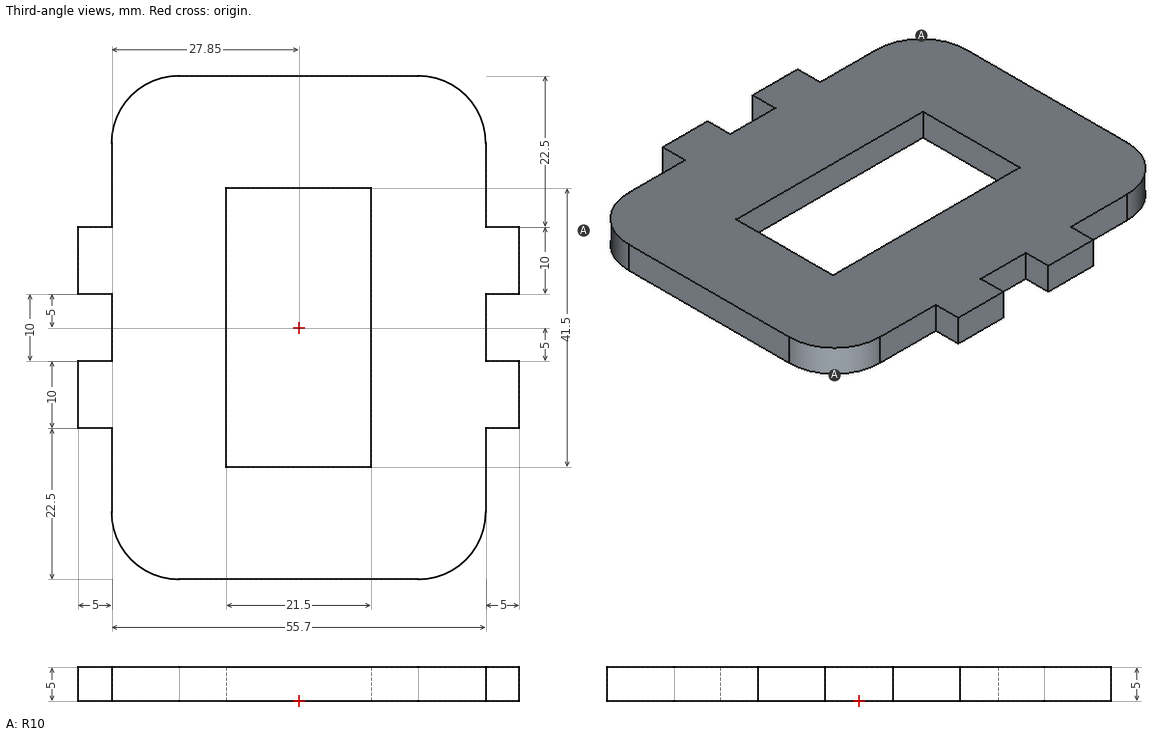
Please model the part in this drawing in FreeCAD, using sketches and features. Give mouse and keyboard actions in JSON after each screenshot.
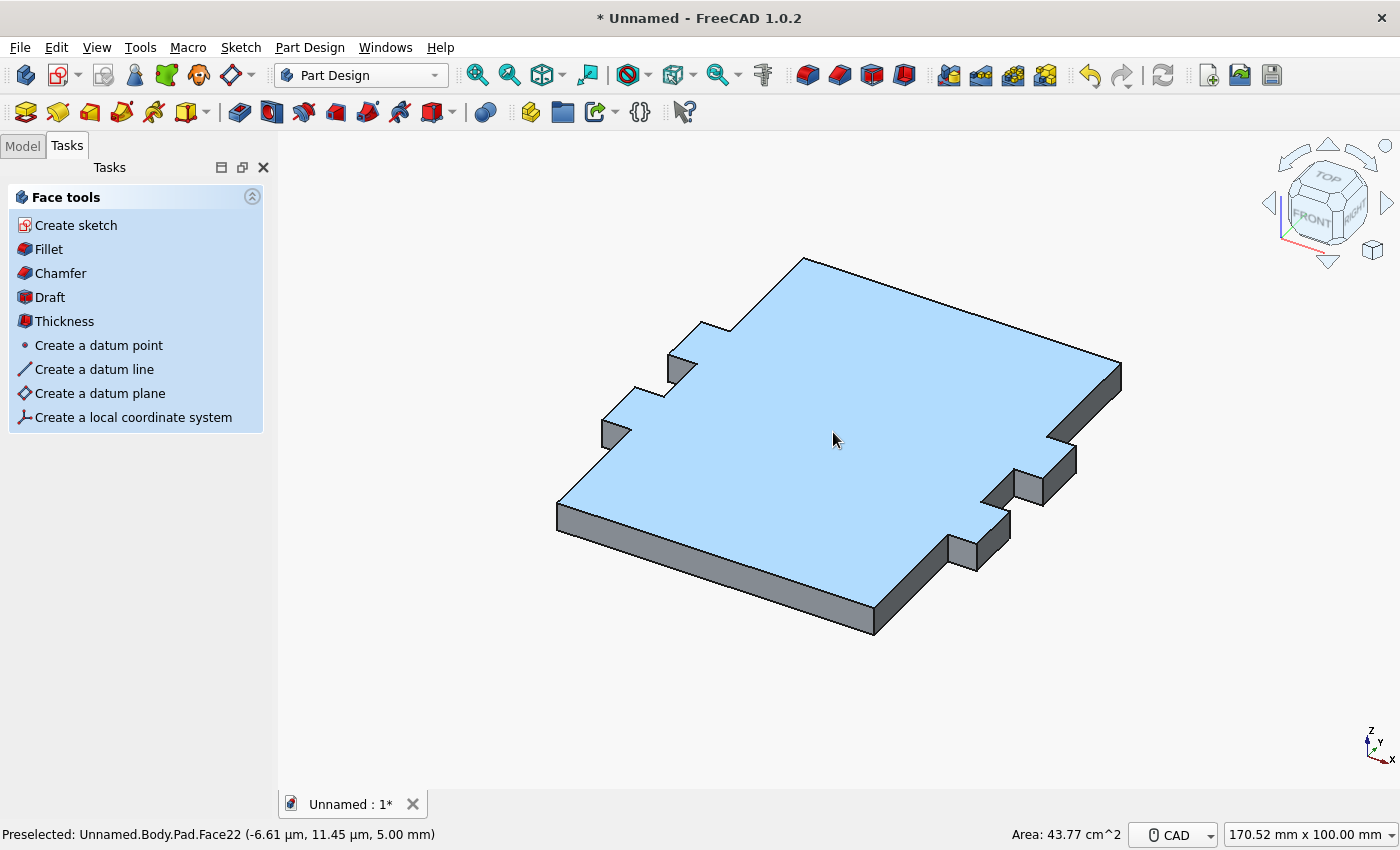
{"action": "left_click", "coordinate": [58, 76]}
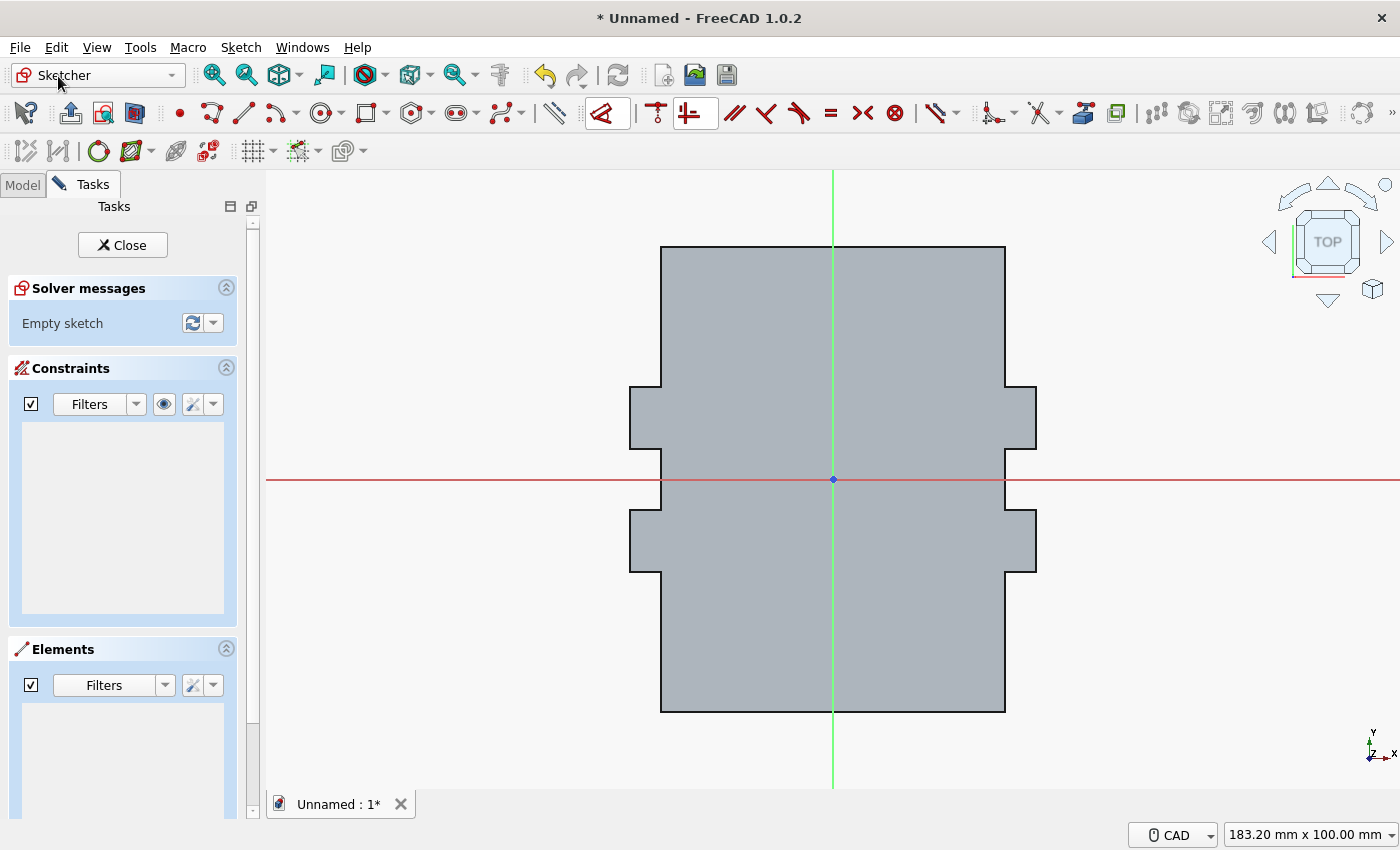
{"action": "scroll", "coordinate": [972, 480], "scroll_direction": "up", "scroll_amount": 2}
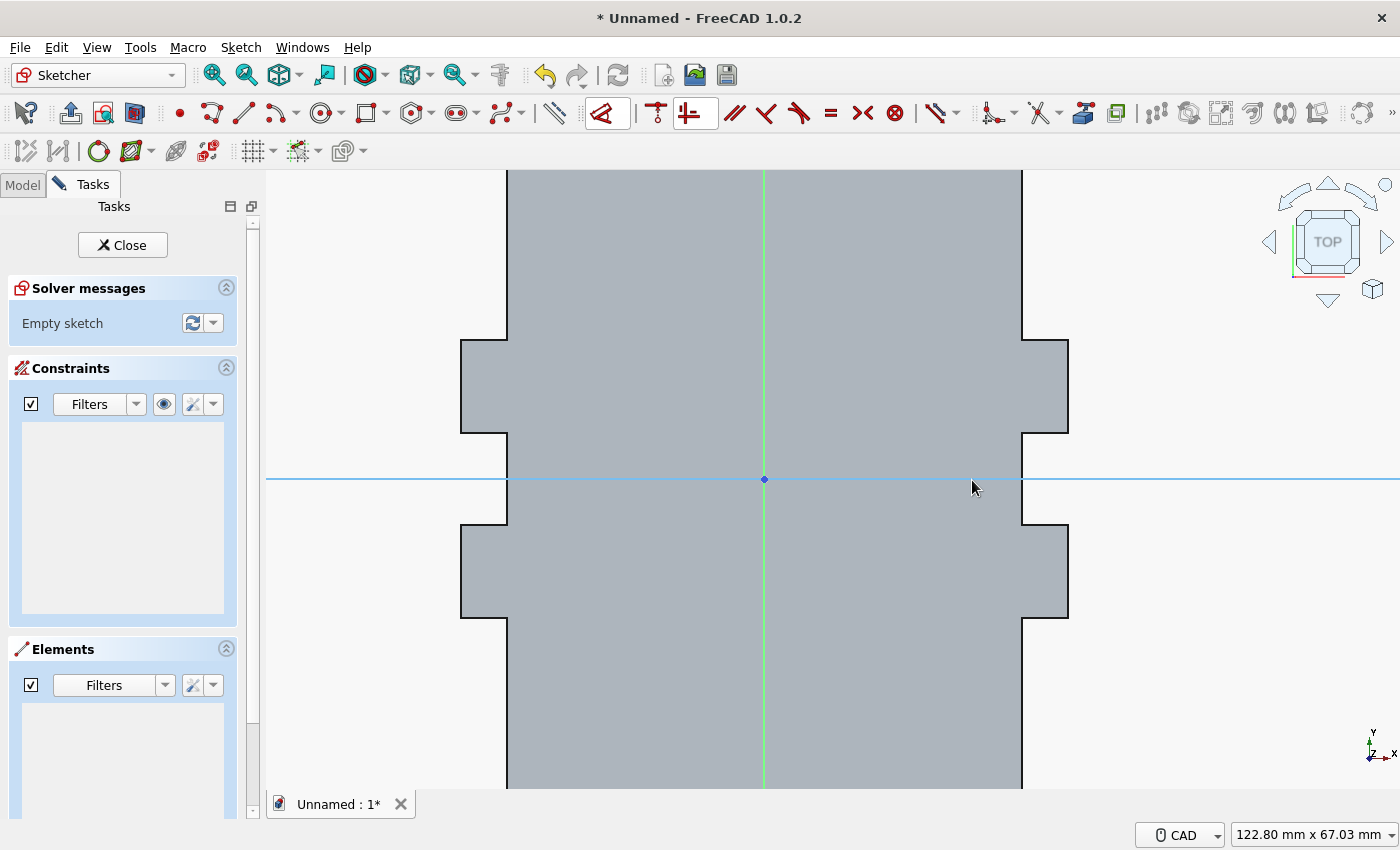
{"action": "left_click", "coordinate": [388, 114]}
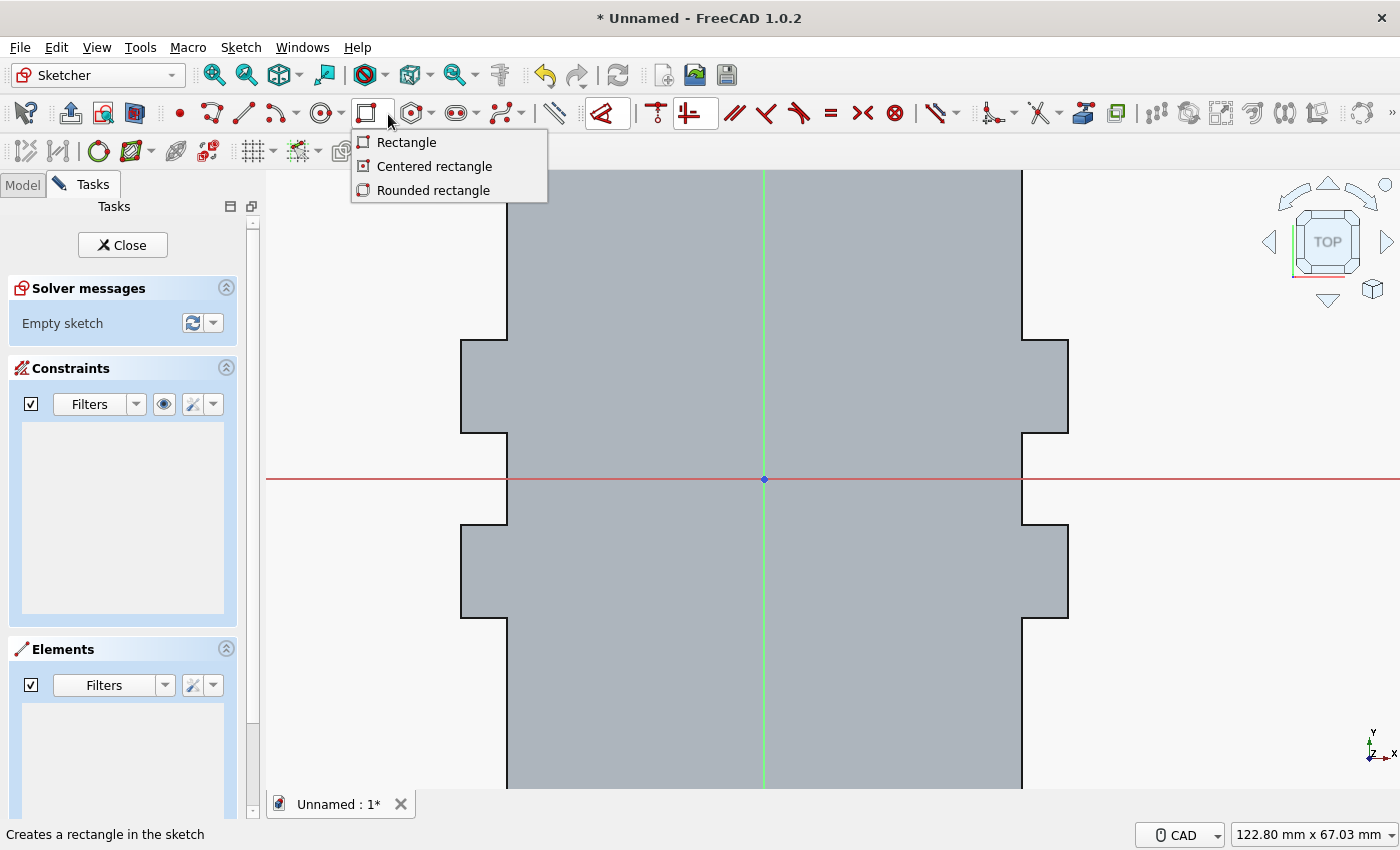
{"action": "left_click", "coordinate": [450, 166]}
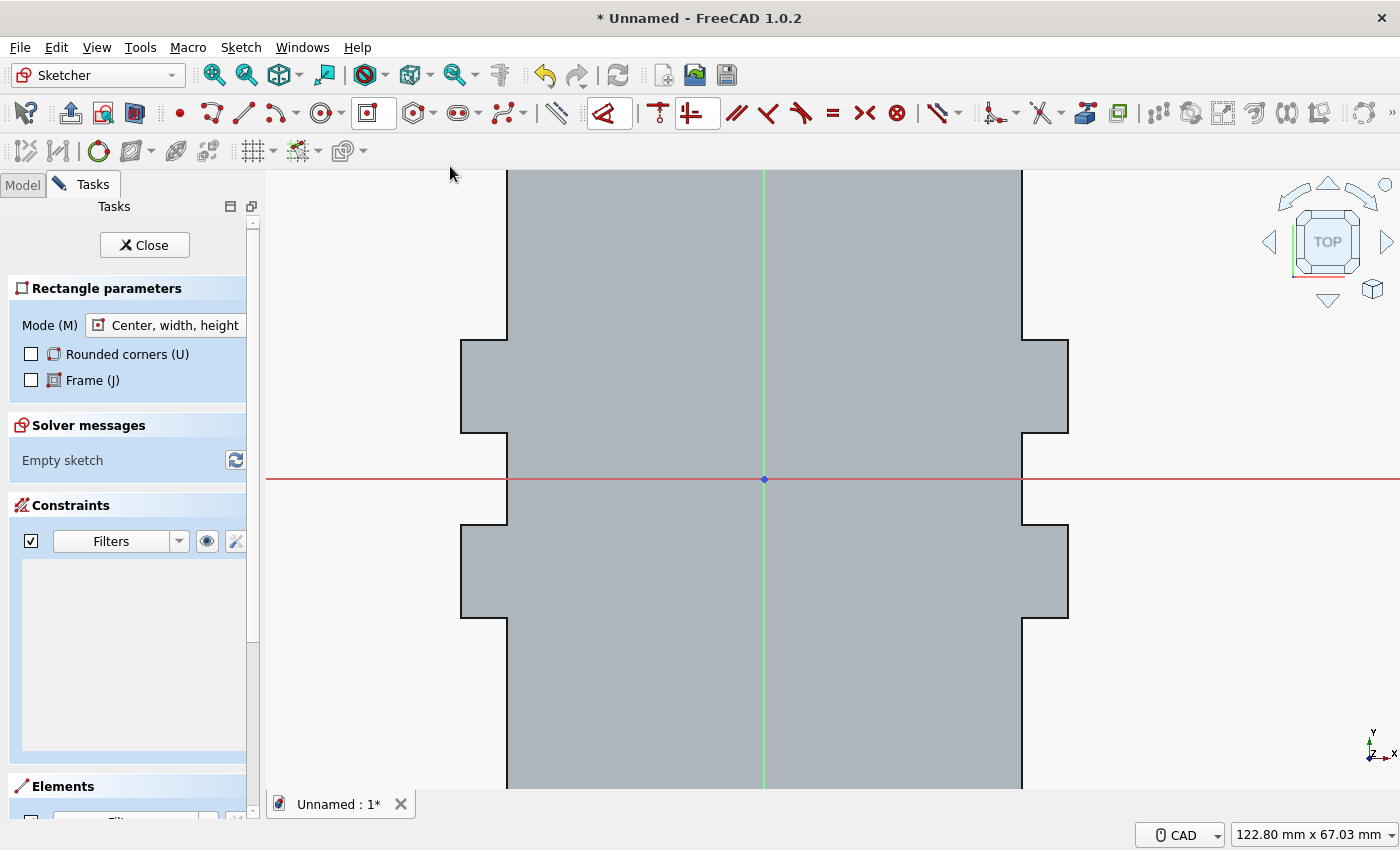
{"action": "left_click", "coordinate": [764, 479]}
{"action": "left_click", "coordinate": [864, 287]}
{"action": "key", "text": "Escape"}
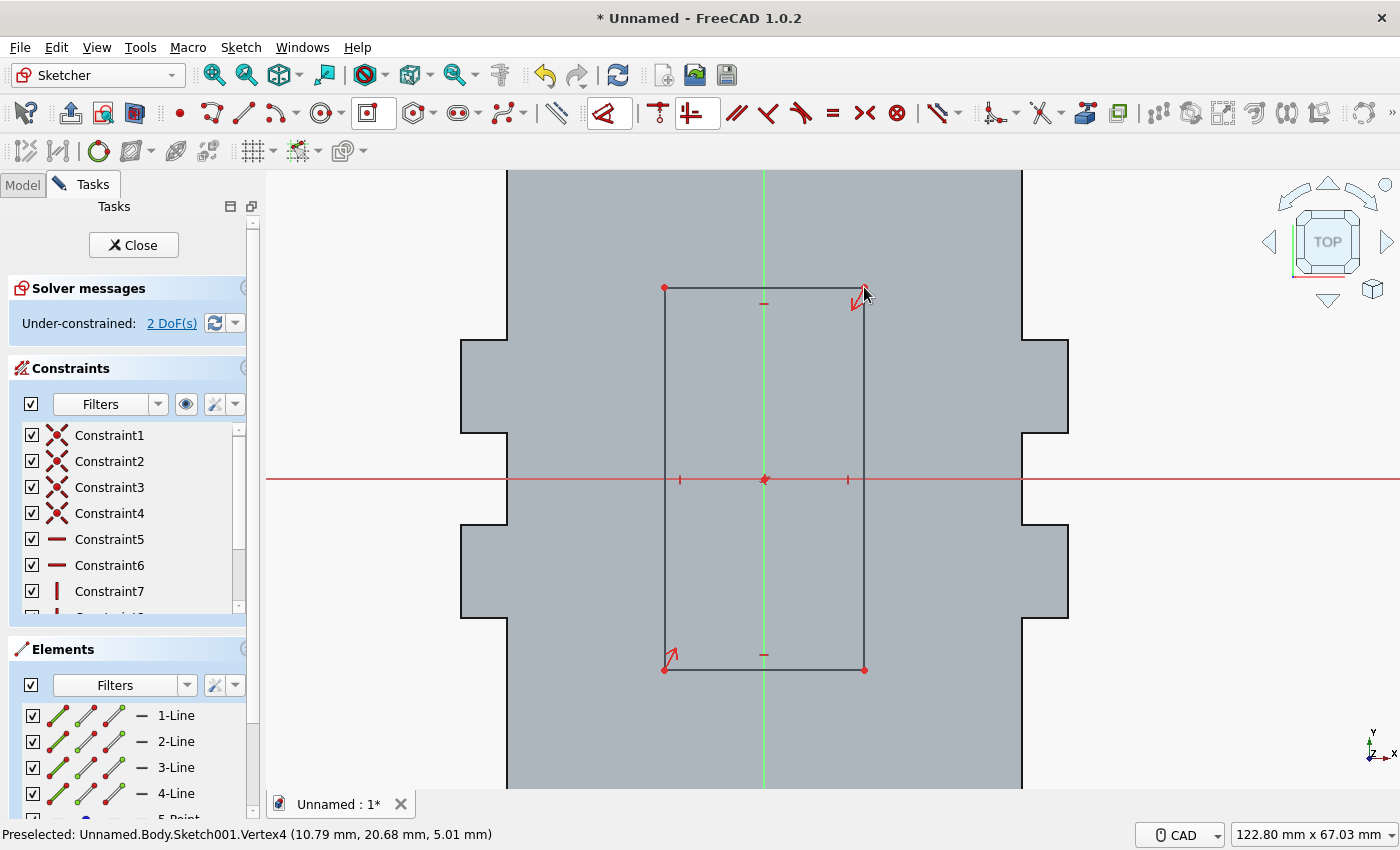
{"action": "left_click", "coordinate": [724, 670]}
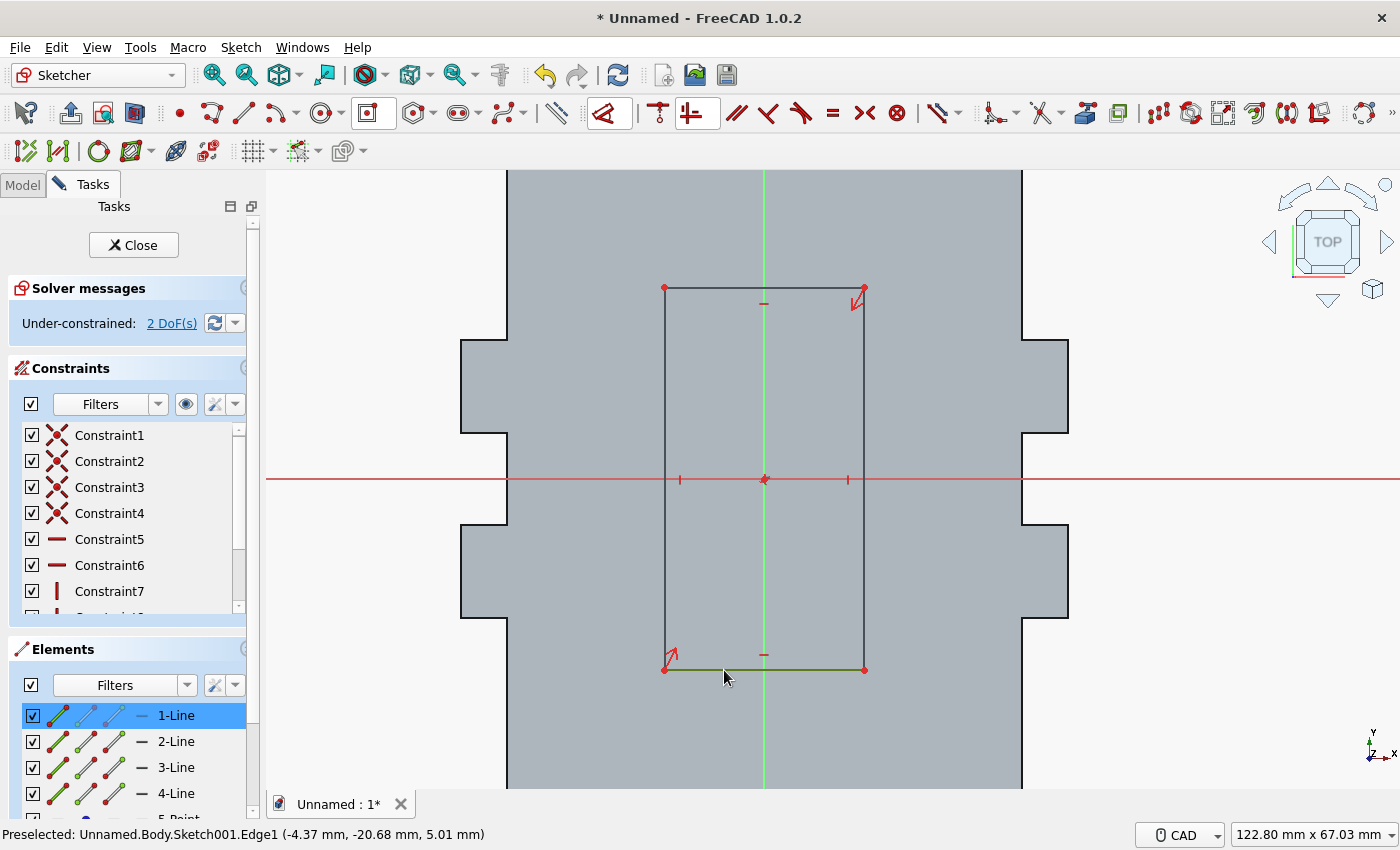
{"action": "left_click", "coordinate": [626, 114]}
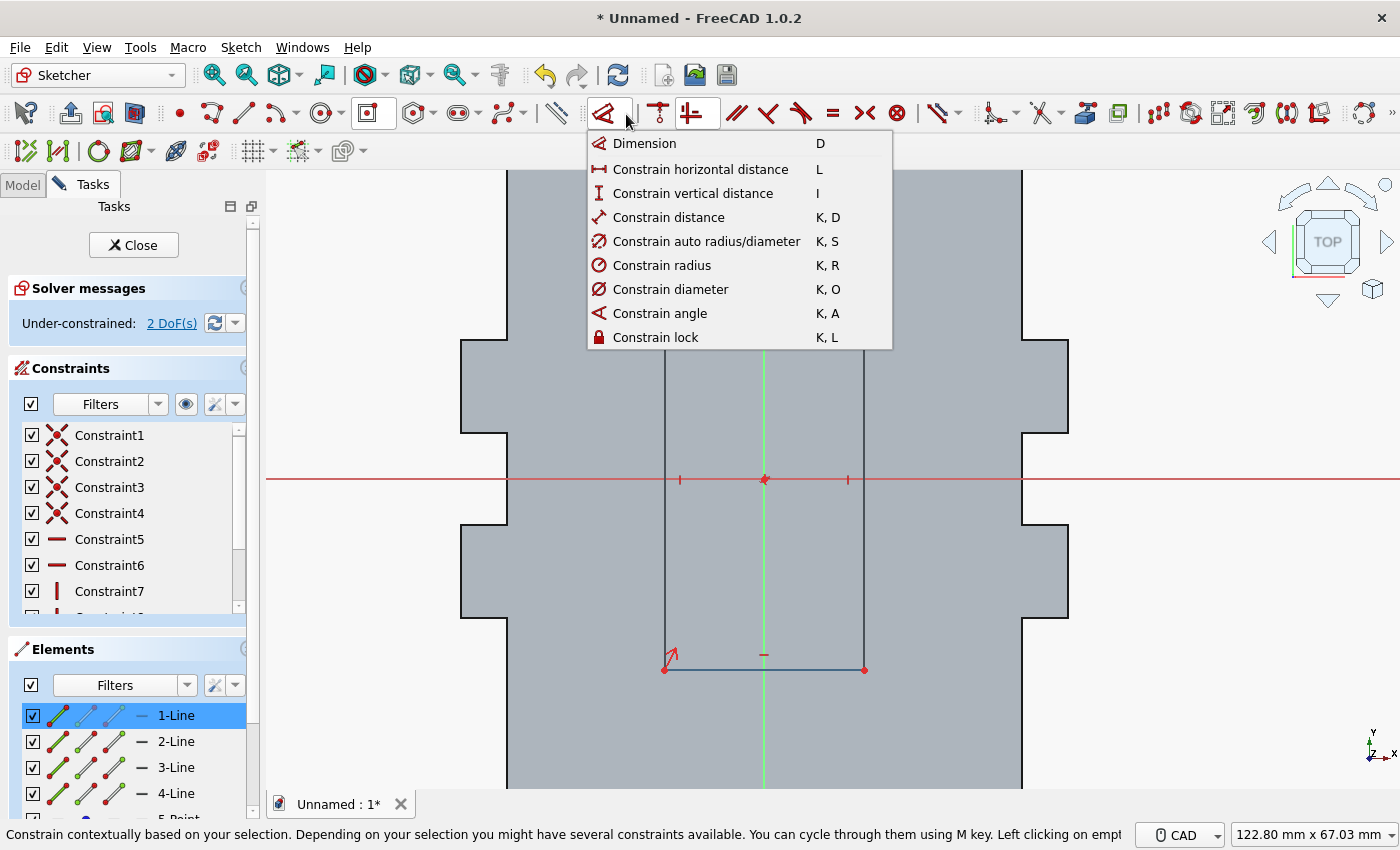
{"action": "left_click", "coordinate": [740, 169]}